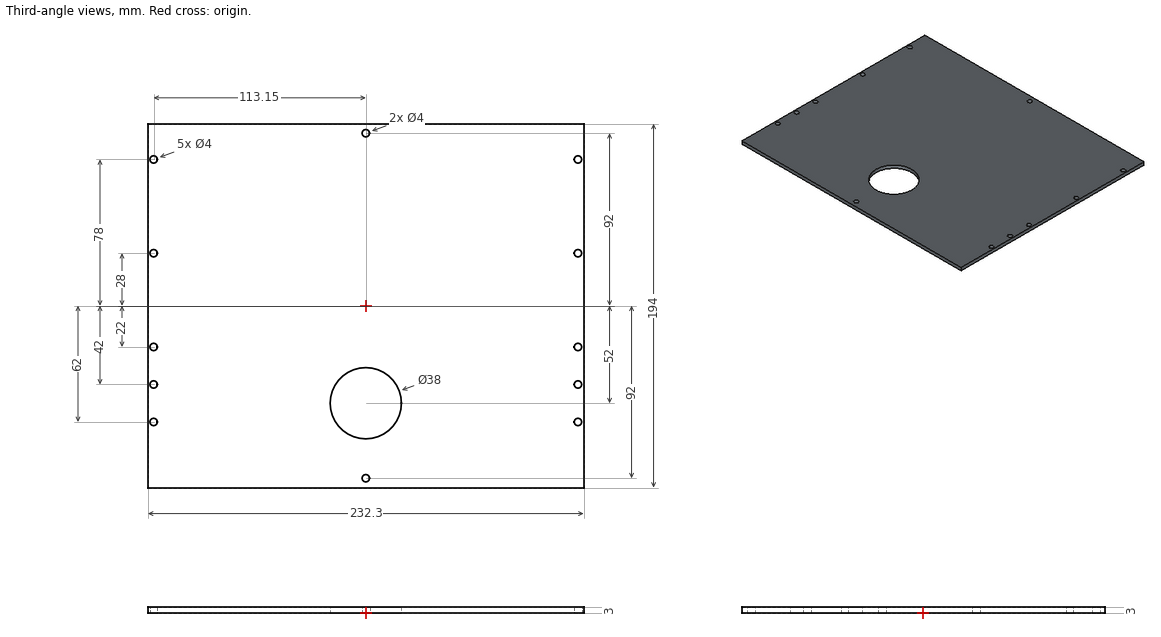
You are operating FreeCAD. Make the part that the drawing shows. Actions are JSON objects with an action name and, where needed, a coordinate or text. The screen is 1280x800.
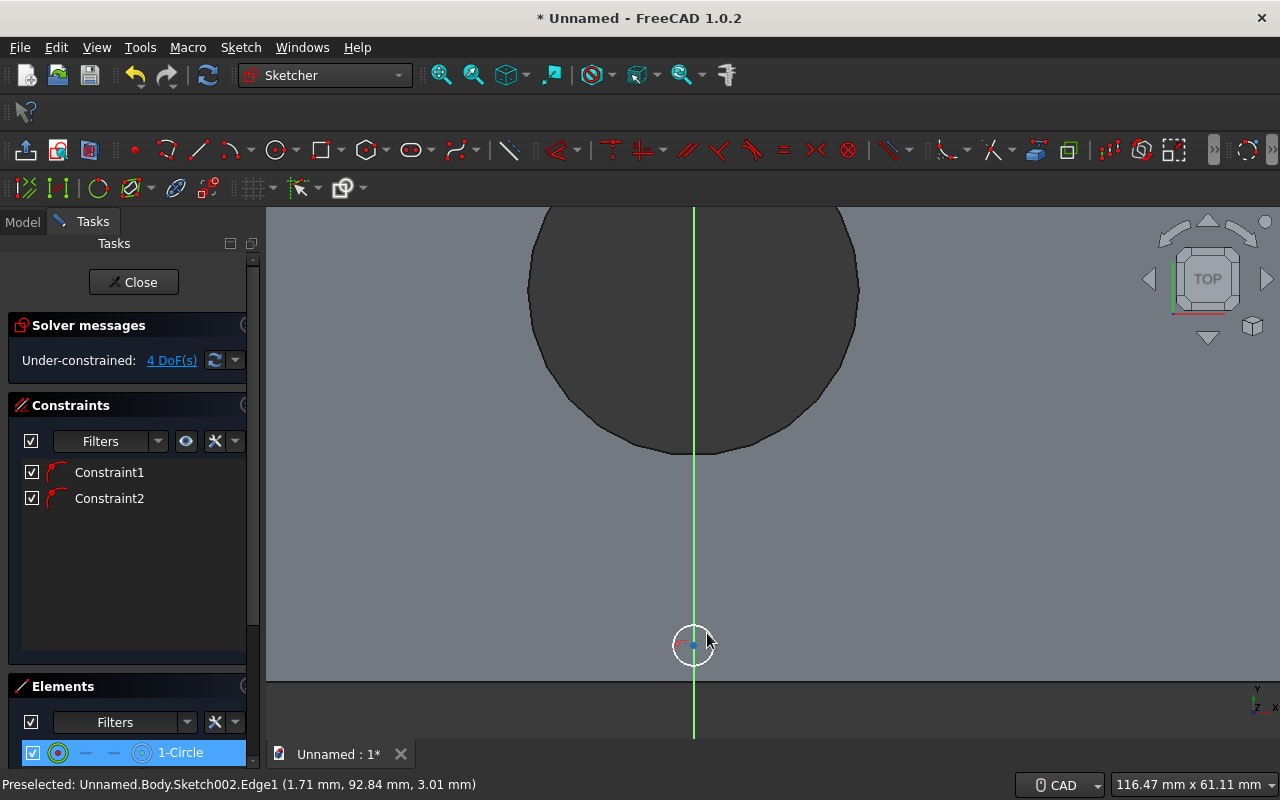
{"action": "left_click", "coordinate": [708, 631]}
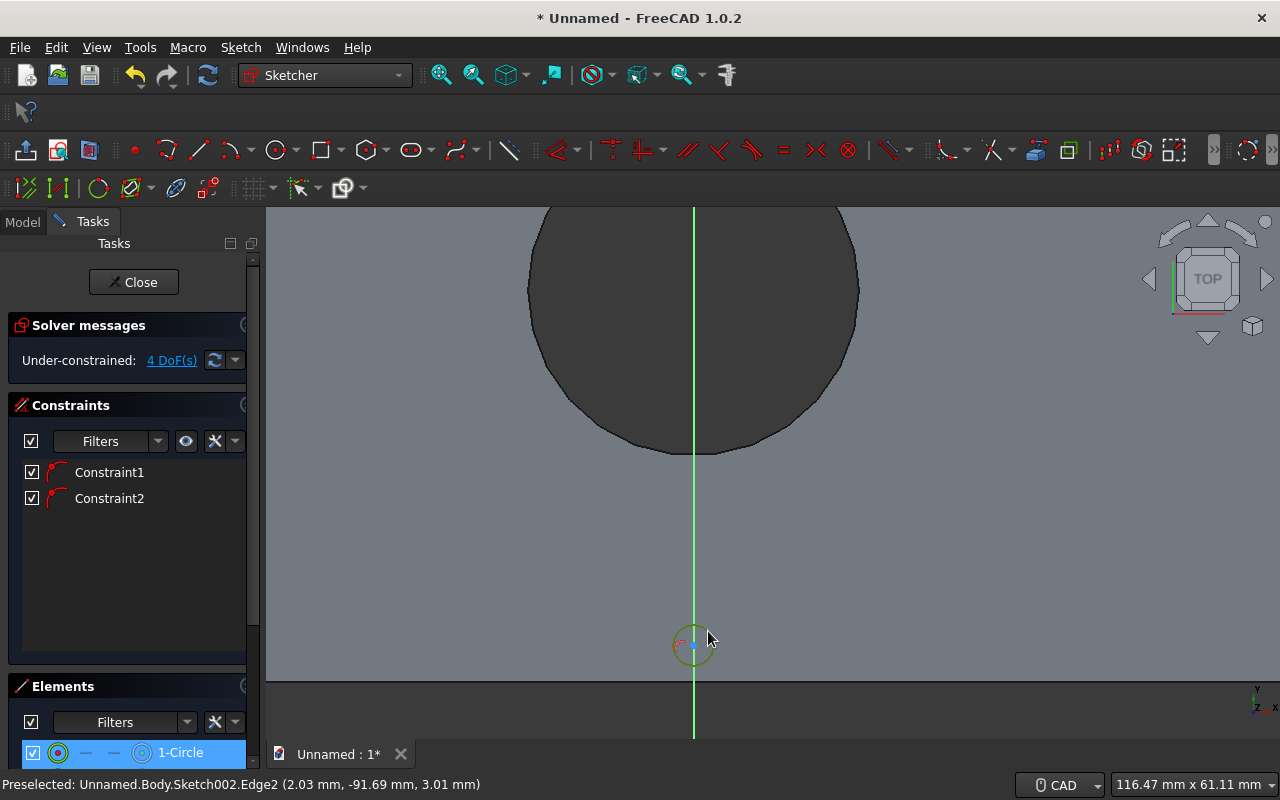
{"action": "key", "text": "e"}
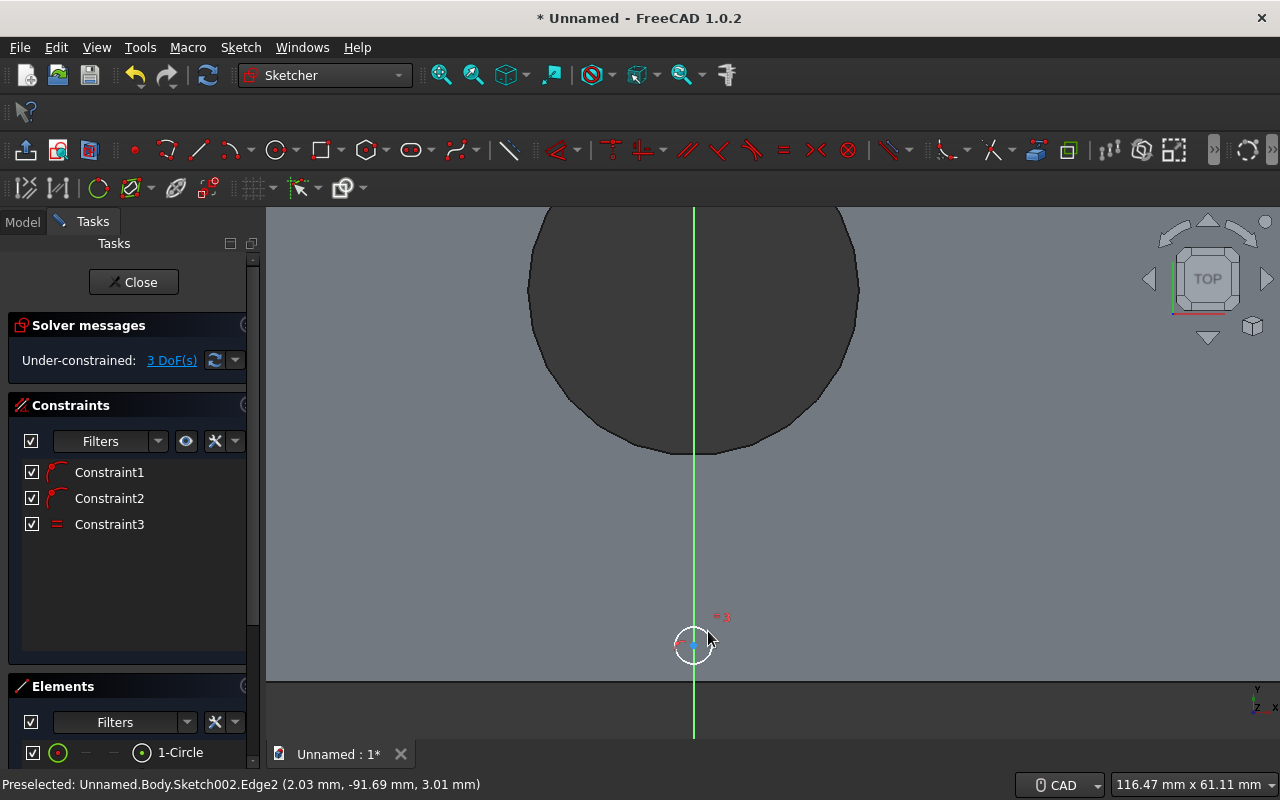
{"action": "left_click", "coordinate": [556, 150]}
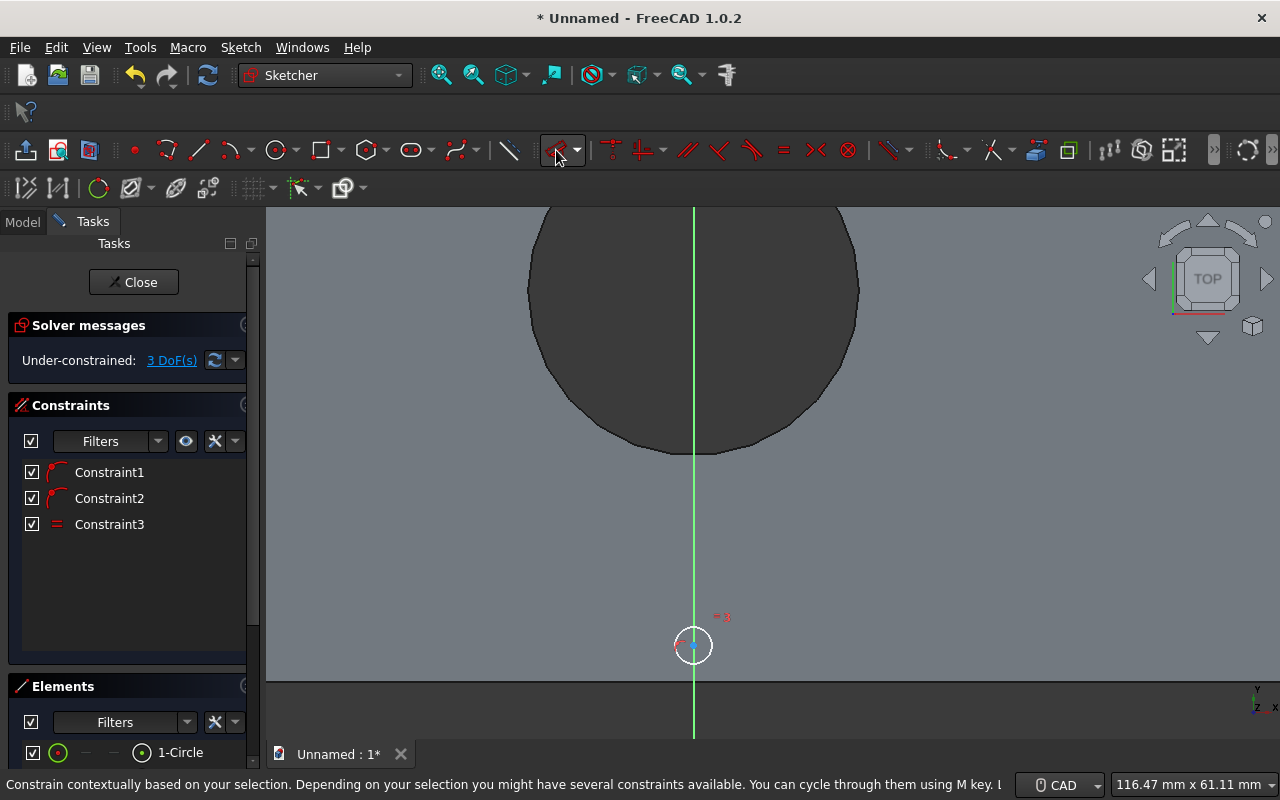
{"action": "scroll", "coordinate": [707, 634], "scroll_direction": "down", "scroll_amount": 8}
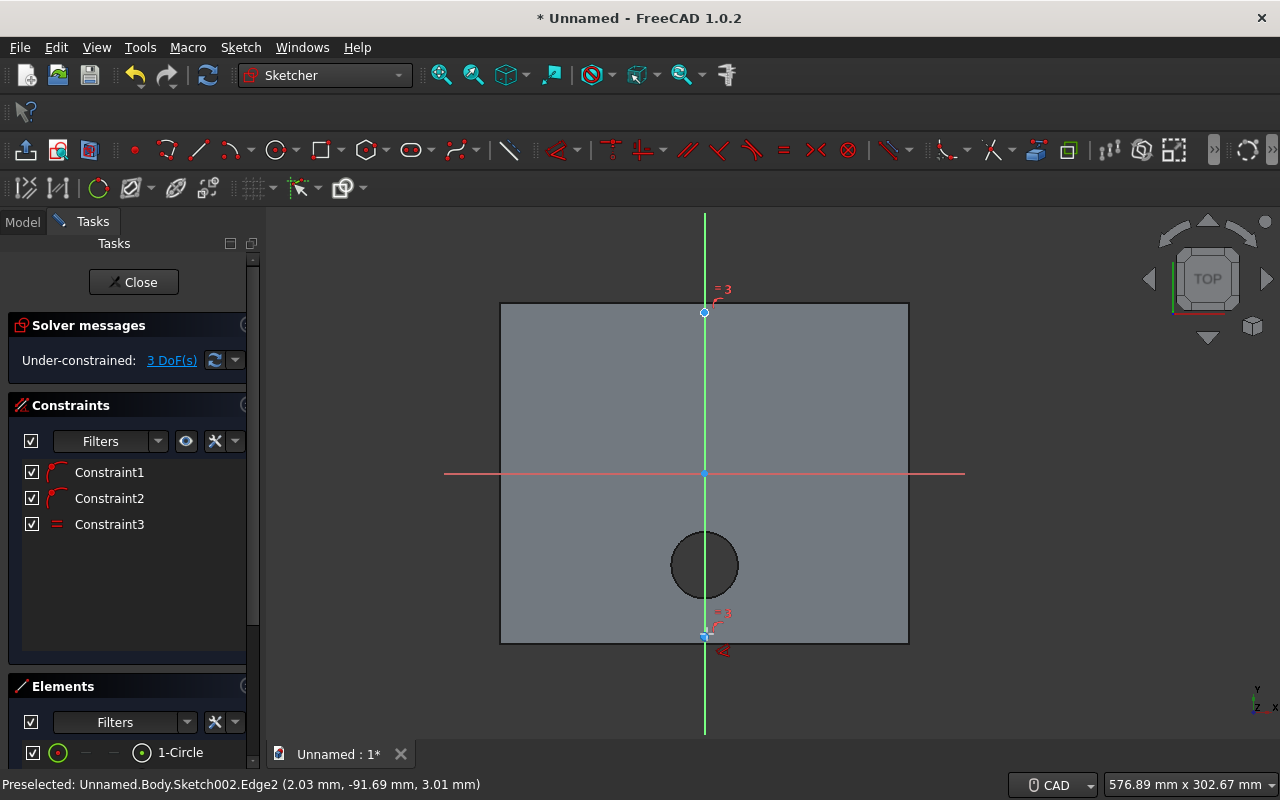
{"action": "scroll", "coordinate": [707, 310], "scroll_direction": "up", "scroll_amount": 9}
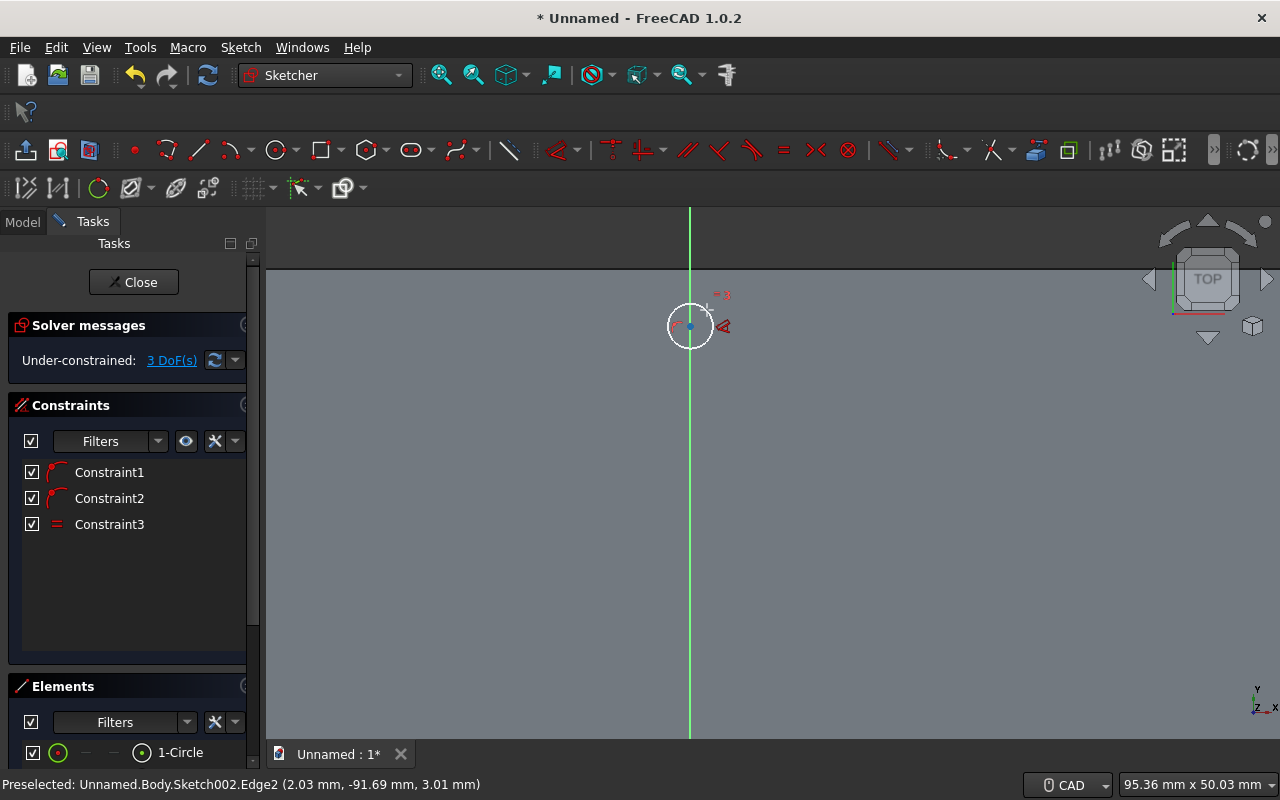
{"action": "left_click", "coordinate": [706, 310]}
{"action": "left_click", "coordinate": [728, 287]}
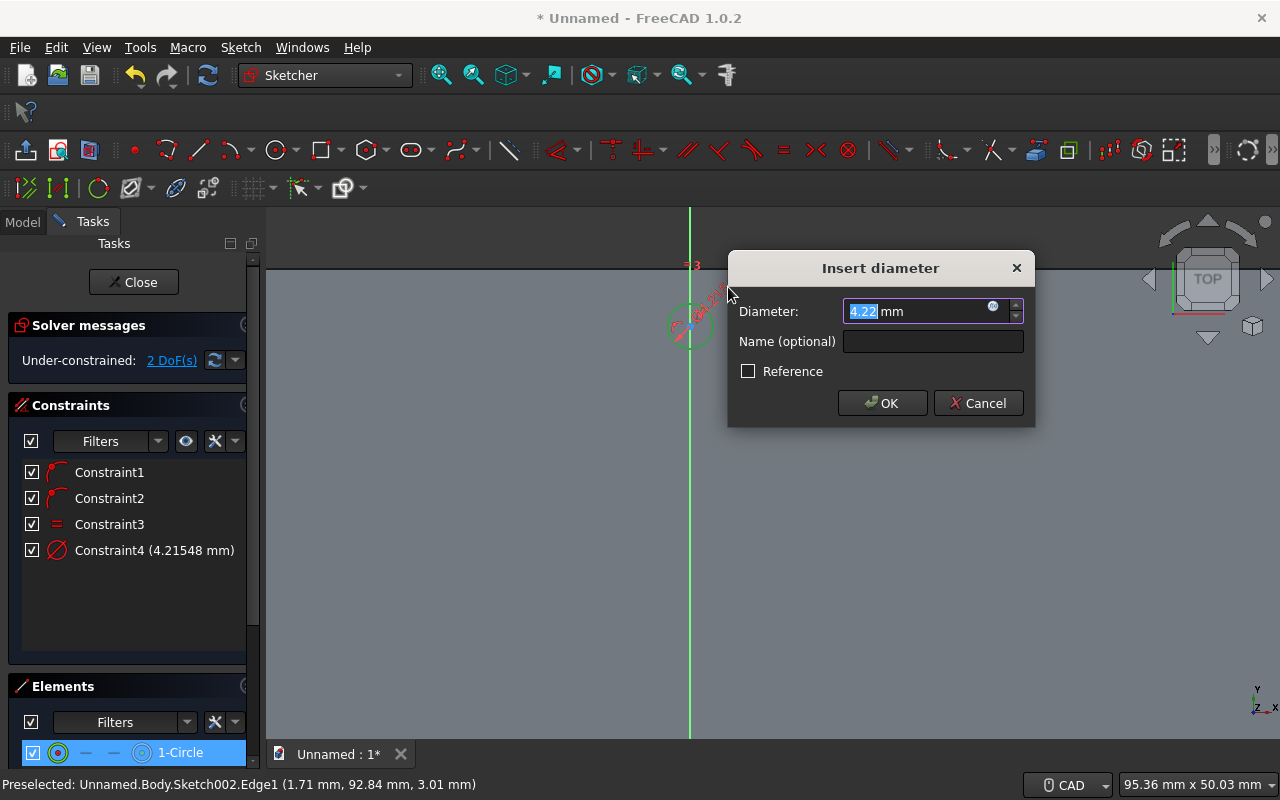
{"action": "type", "text": "4"}
{"action": "key", "text": "Return"}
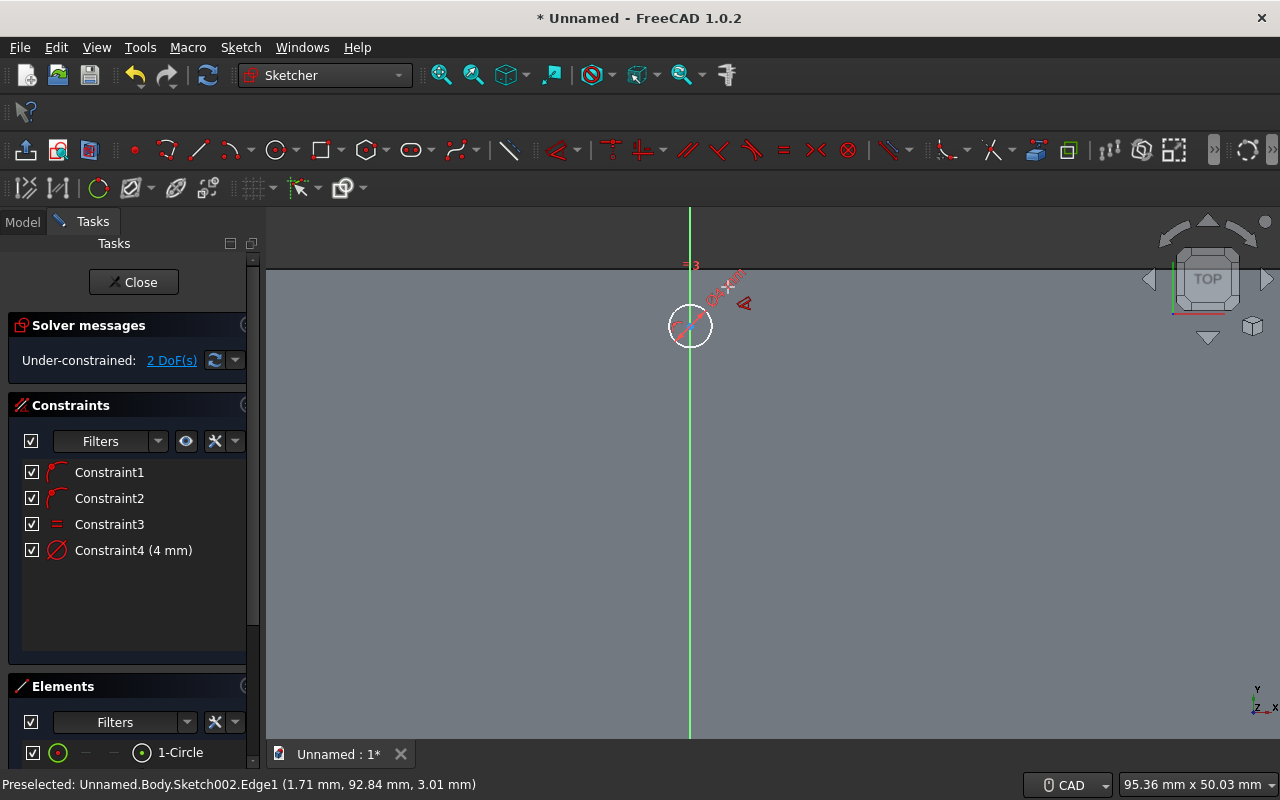
{"action": "scroll", "coordinate": [707, 309], "scroll_direction": "down", "scroll_amount": 9}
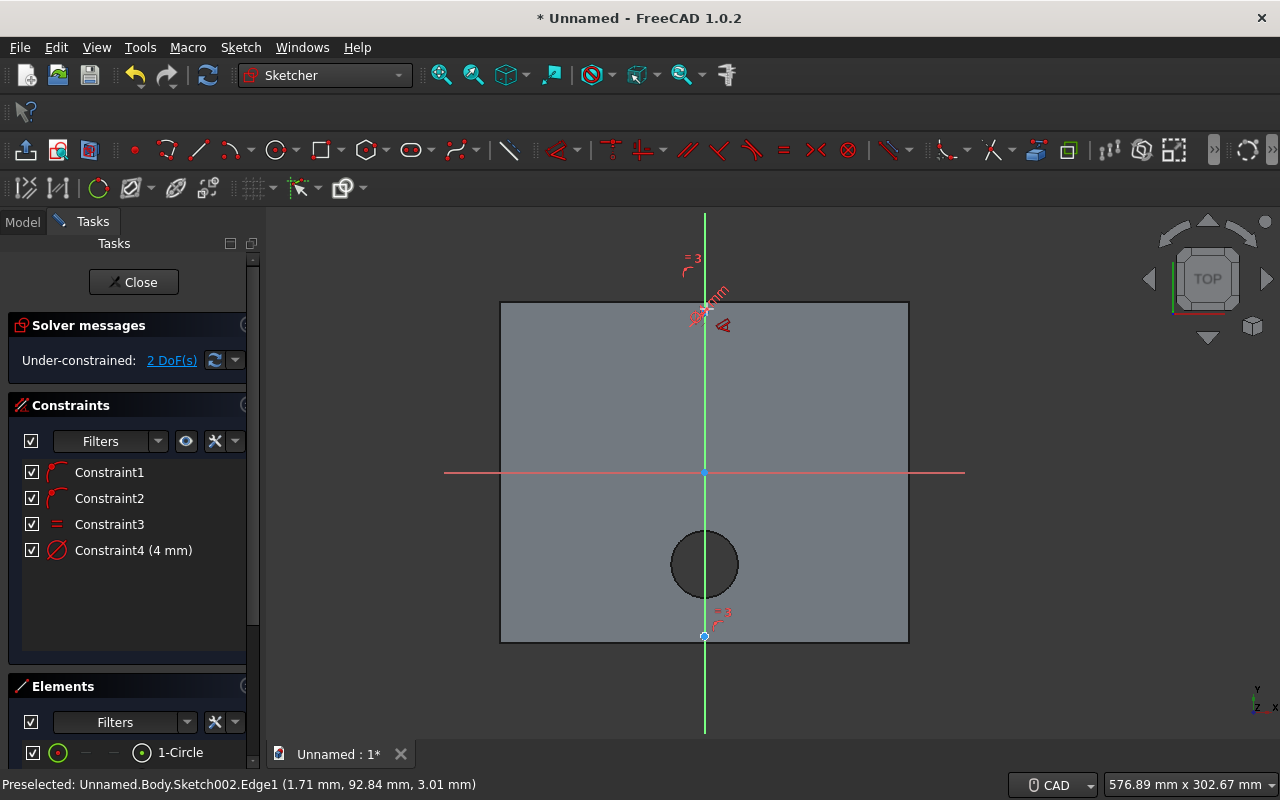
{"action": "left_click", "coordinate": [705, 312]}
{"action": "left_click", "coordinate": [739, 392]}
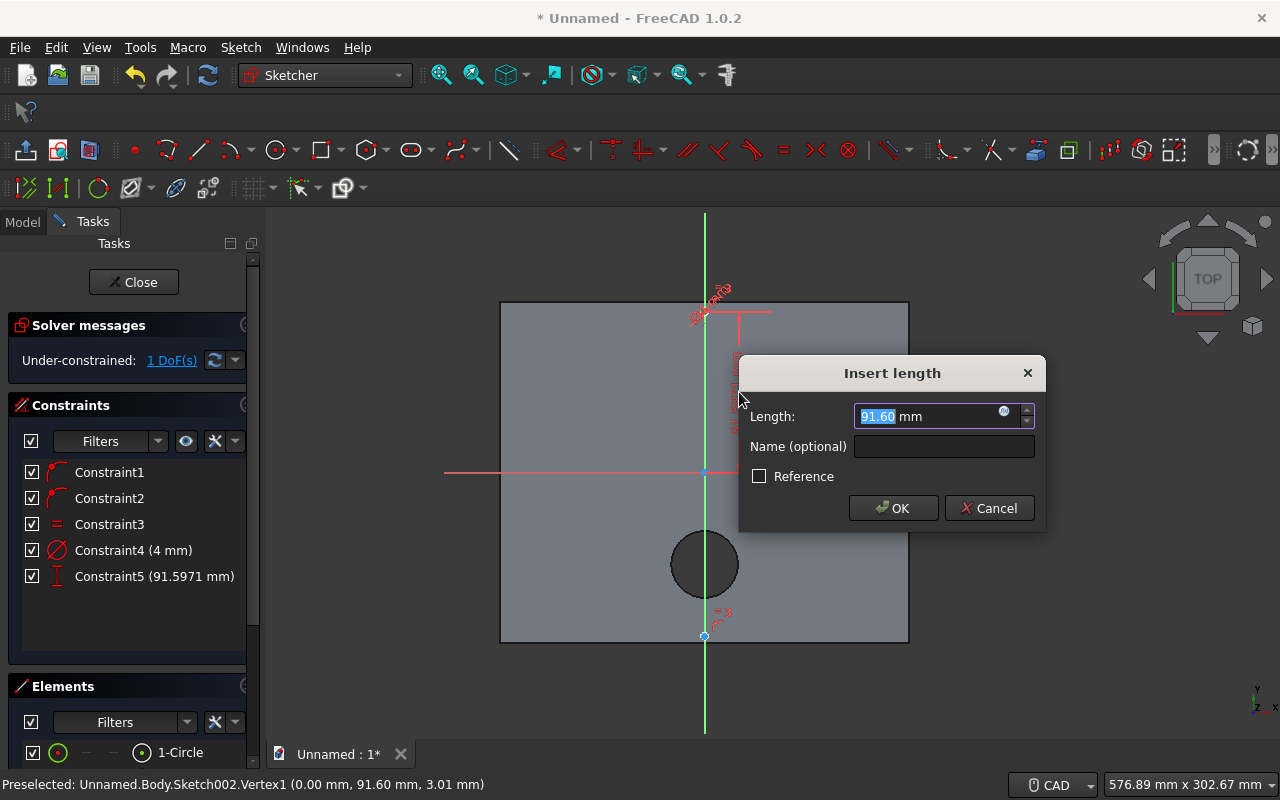
{"action": "type", "text": "92"}
{"action": "key", "text": "Return"}